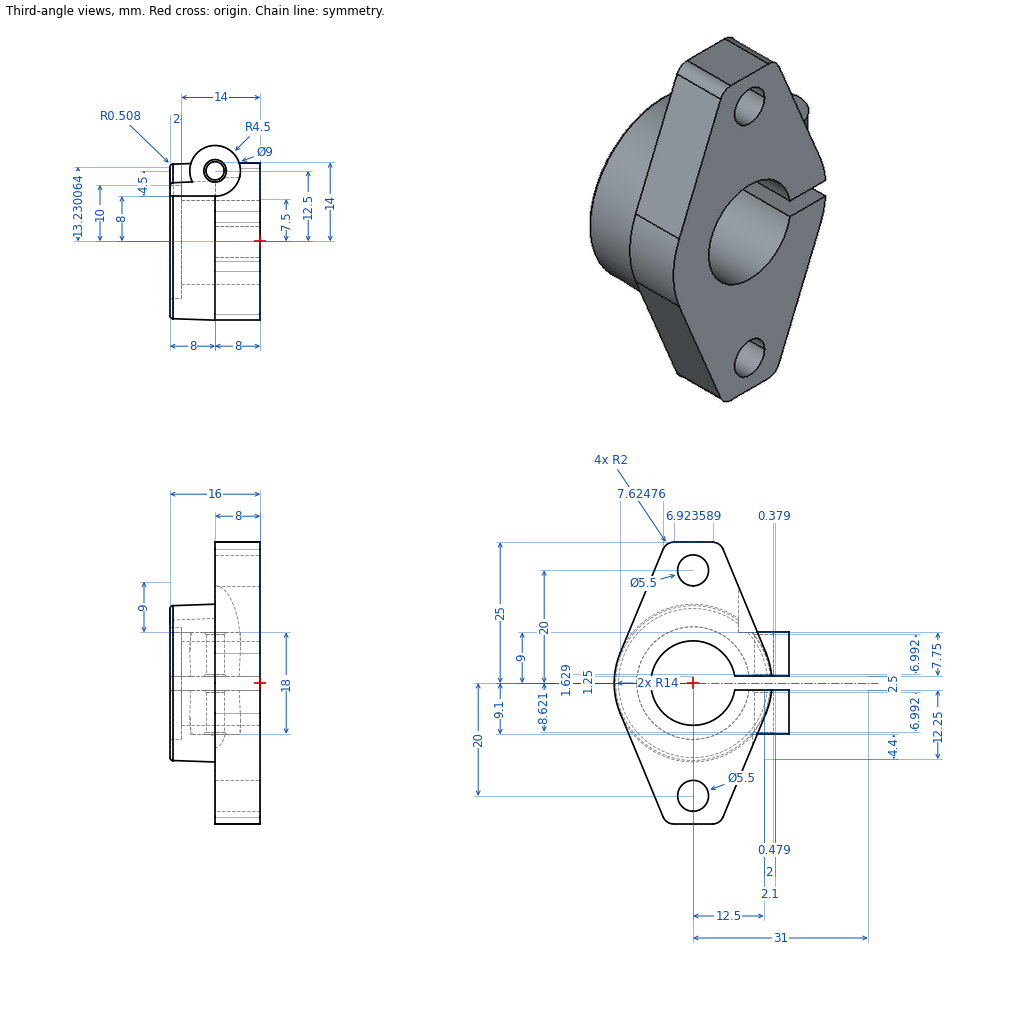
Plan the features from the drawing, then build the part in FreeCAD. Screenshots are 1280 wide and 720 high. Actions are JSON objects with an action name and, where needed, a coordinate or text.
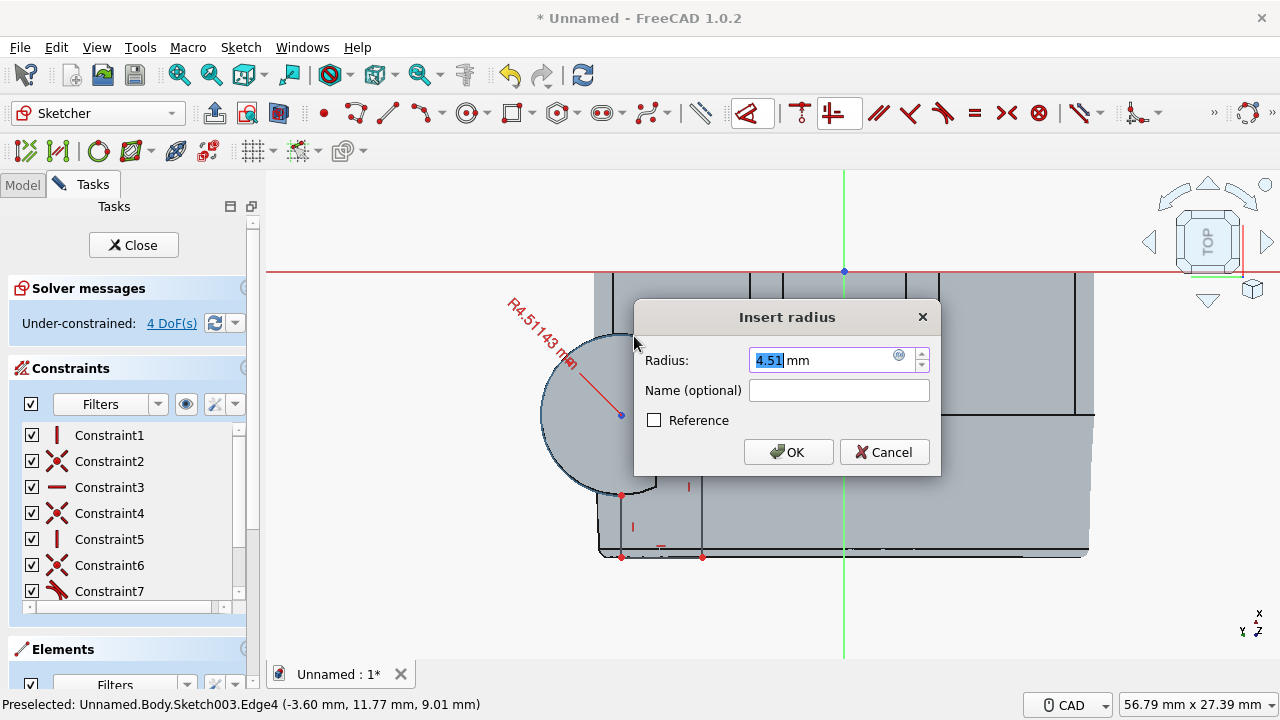
{"action": "type", "text": "4.5"}
{"action": "key", "text": "Return"}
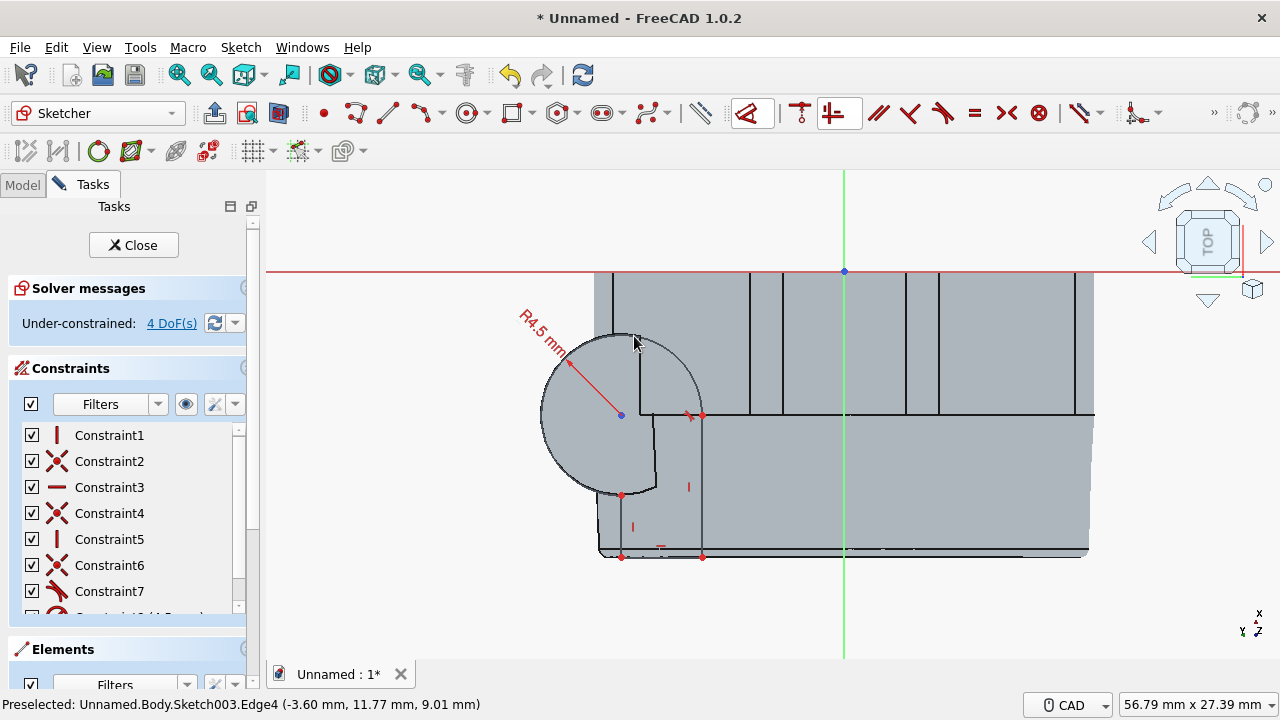
{"action": "left_click", "coordinate": [702, 515]}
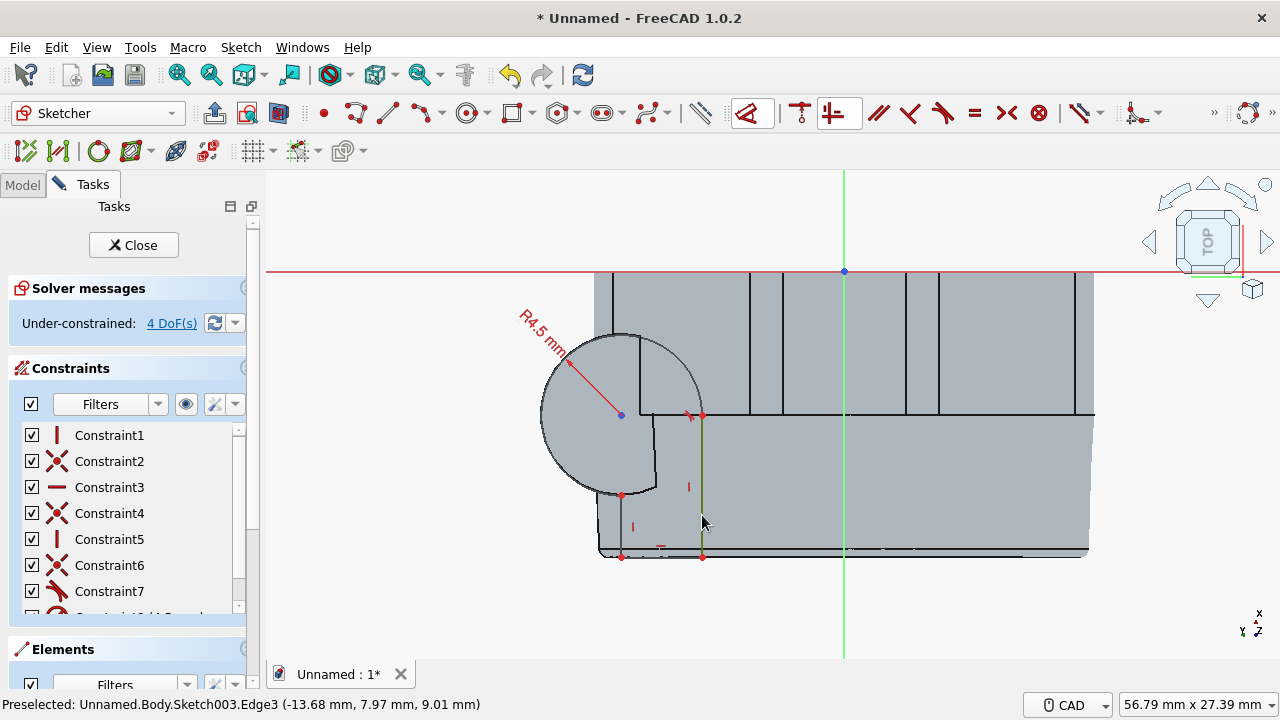
{"action": "left_click", "coordinate": [768, 114]}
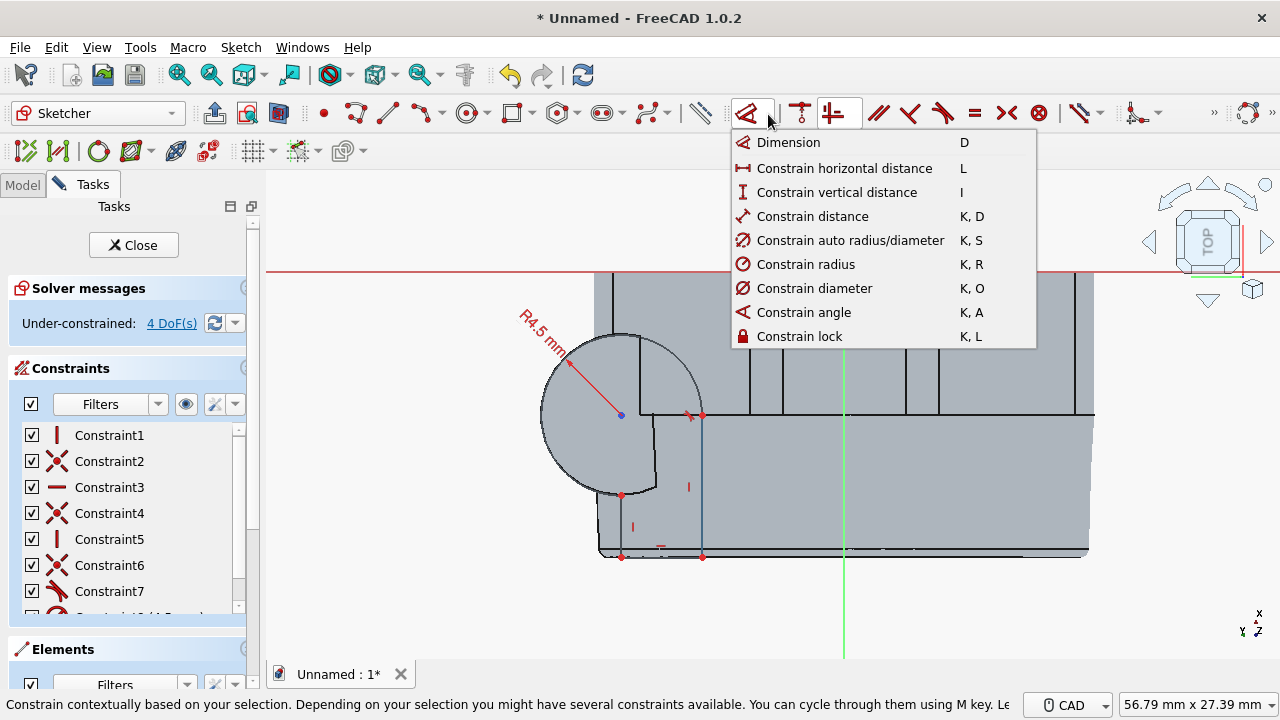
{"action": "left_click", "coordinate": [884, 192]}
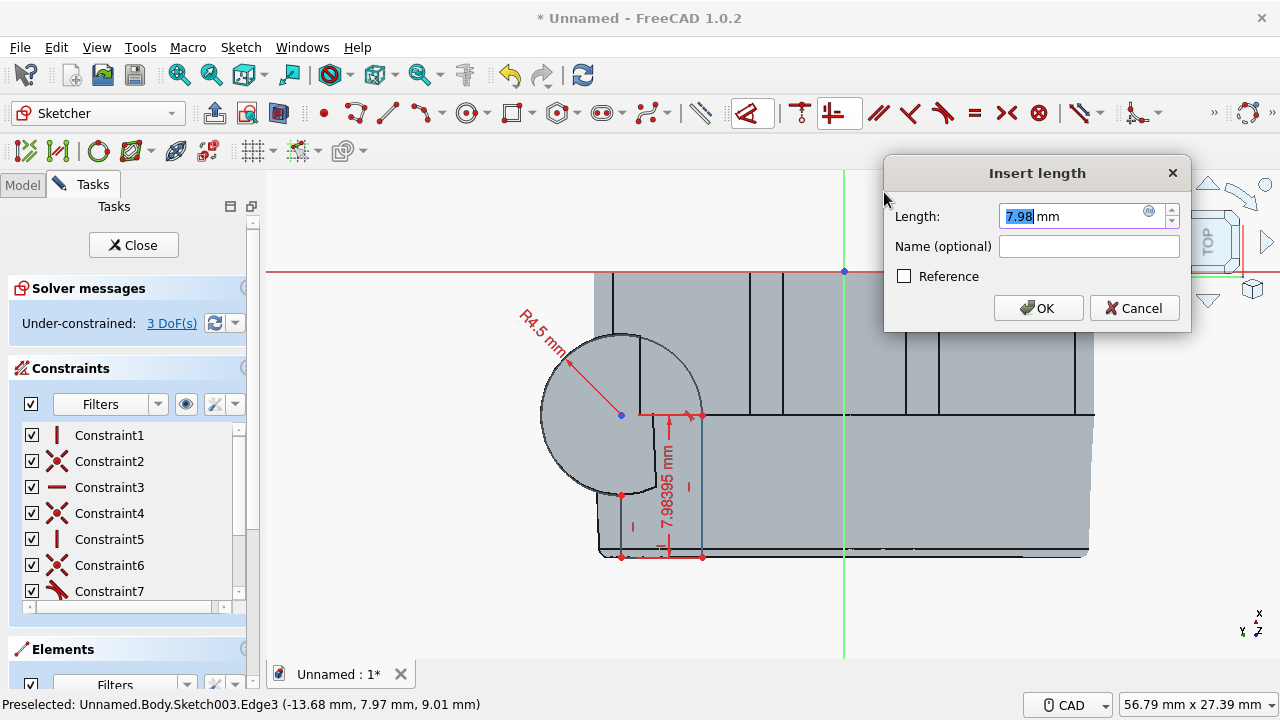
{"action": "type", "text": "8"}
{"action": "key", "text": "Return"}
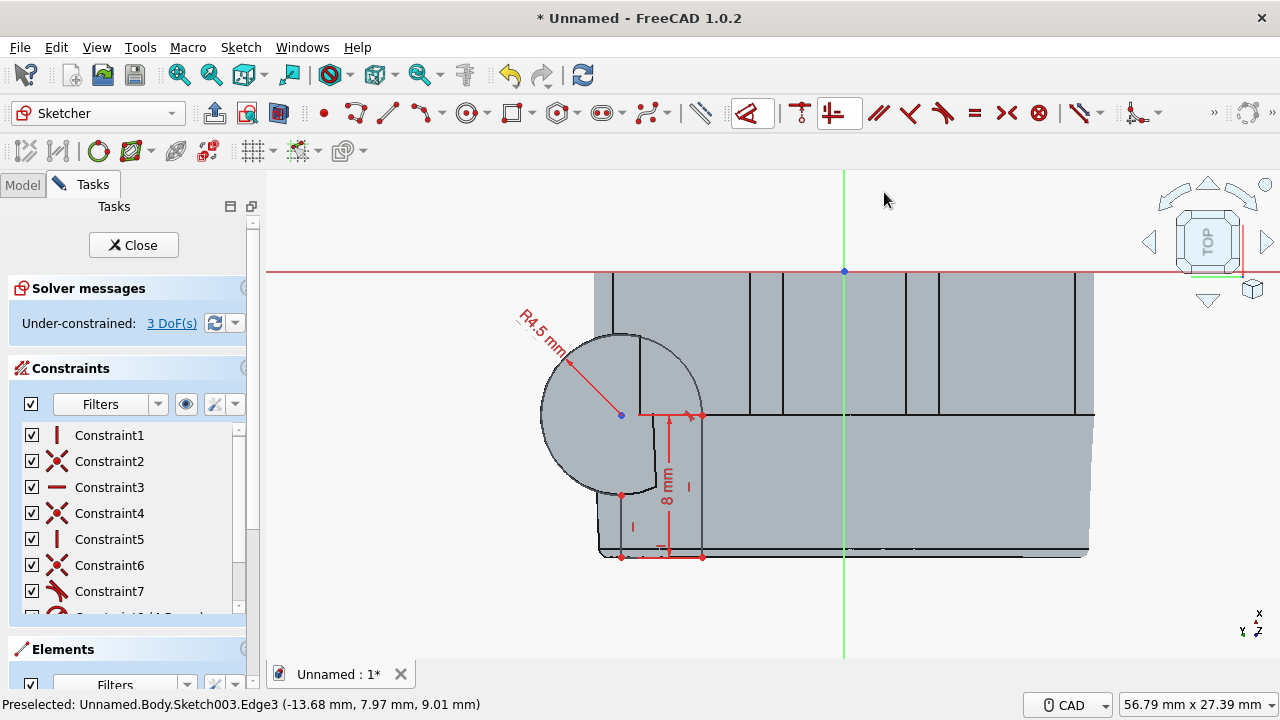
{"action": "left_click", "coordinate": [702, 558]}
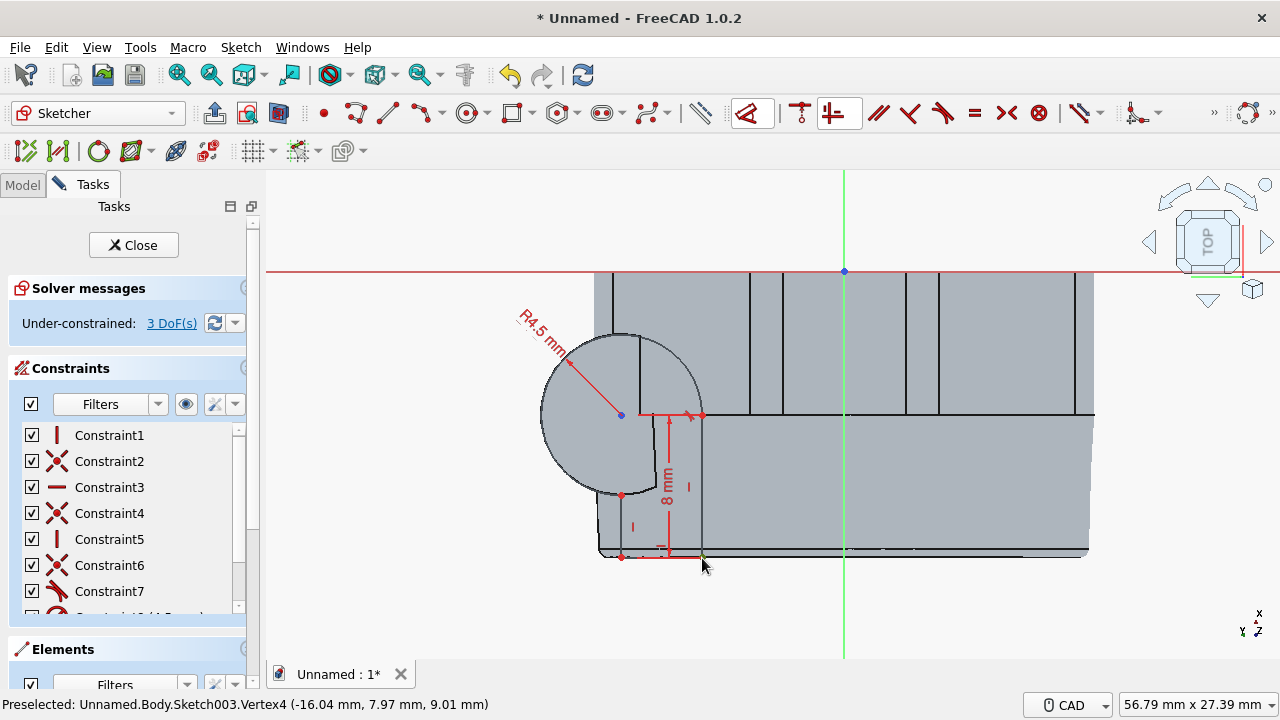
{"action": "left_click", "coordinate": [768, 114]}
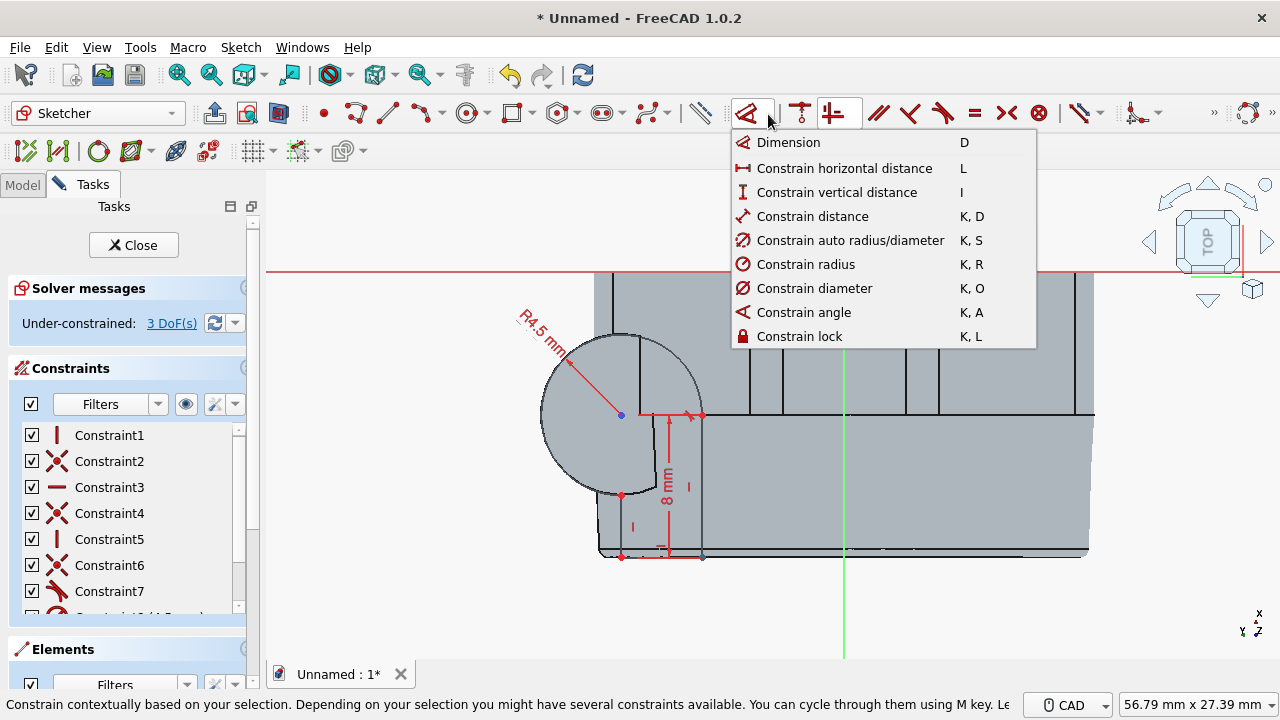
{"action": "left_click", "coordinate": [884, 168]}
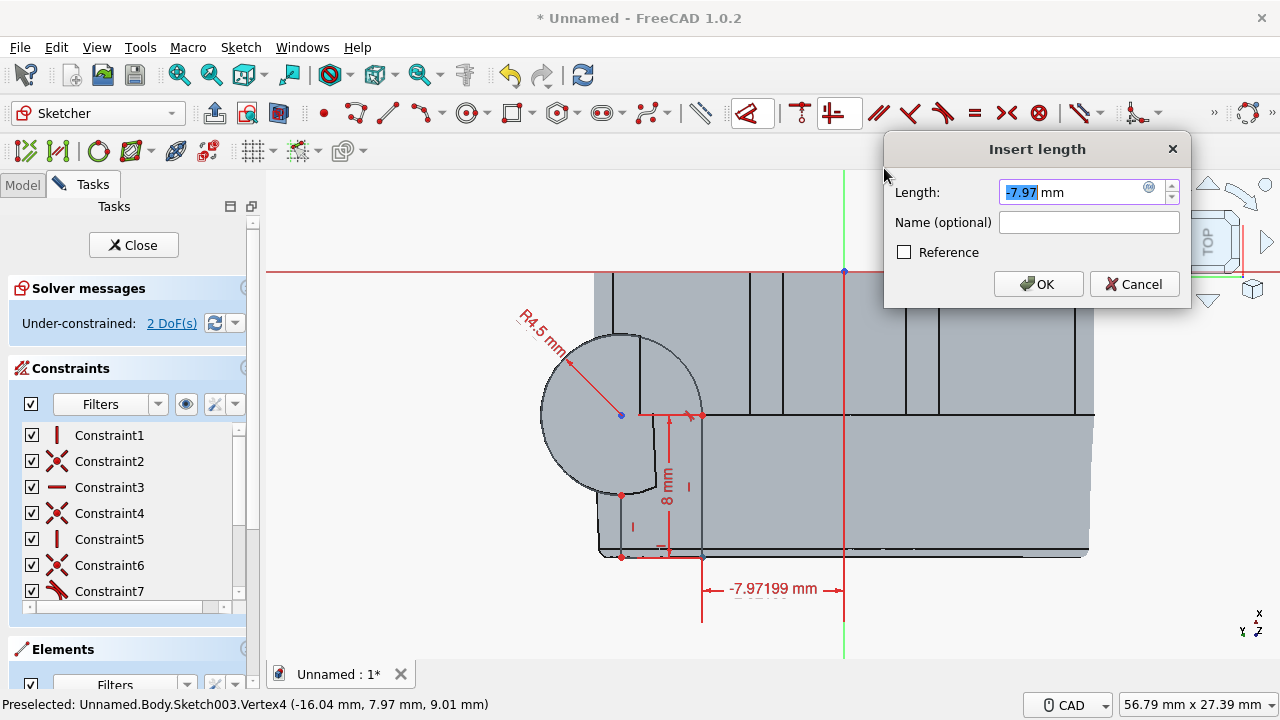
{"action": "type", "text": "-8"}
{"action": "key", "text": "Return"}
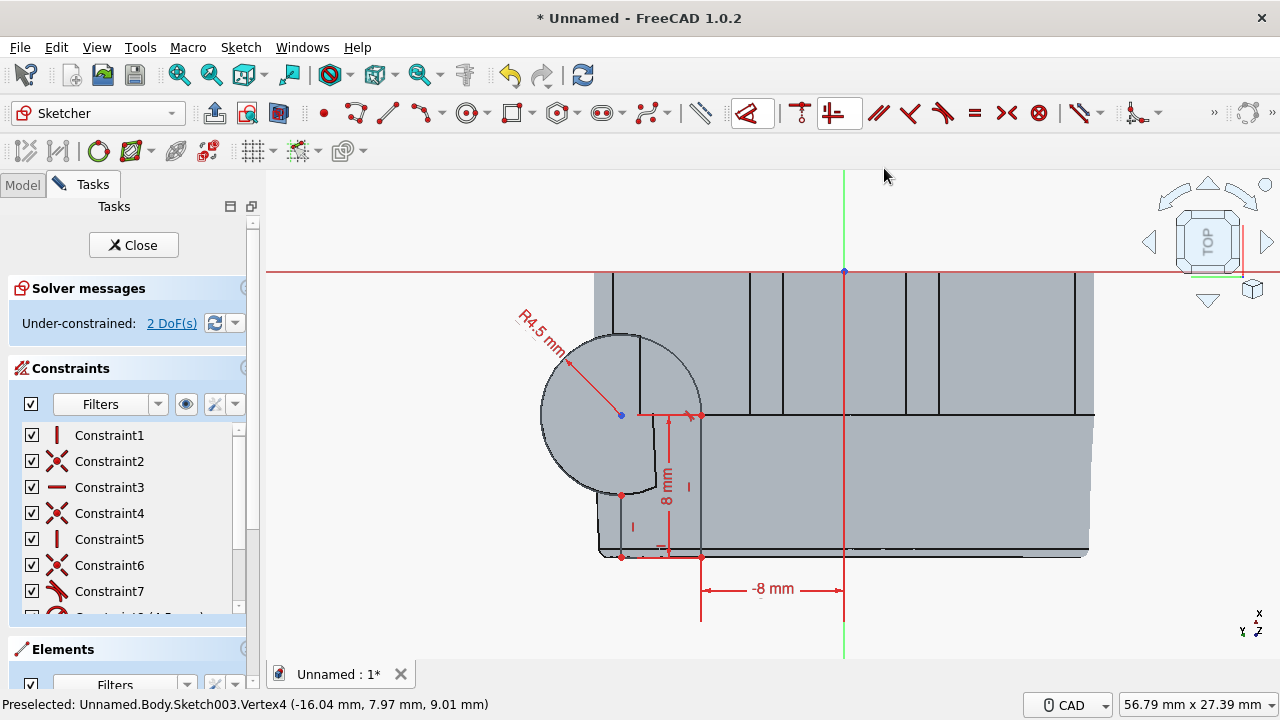
{"action": "left_click", "coordinate": [702, 415]}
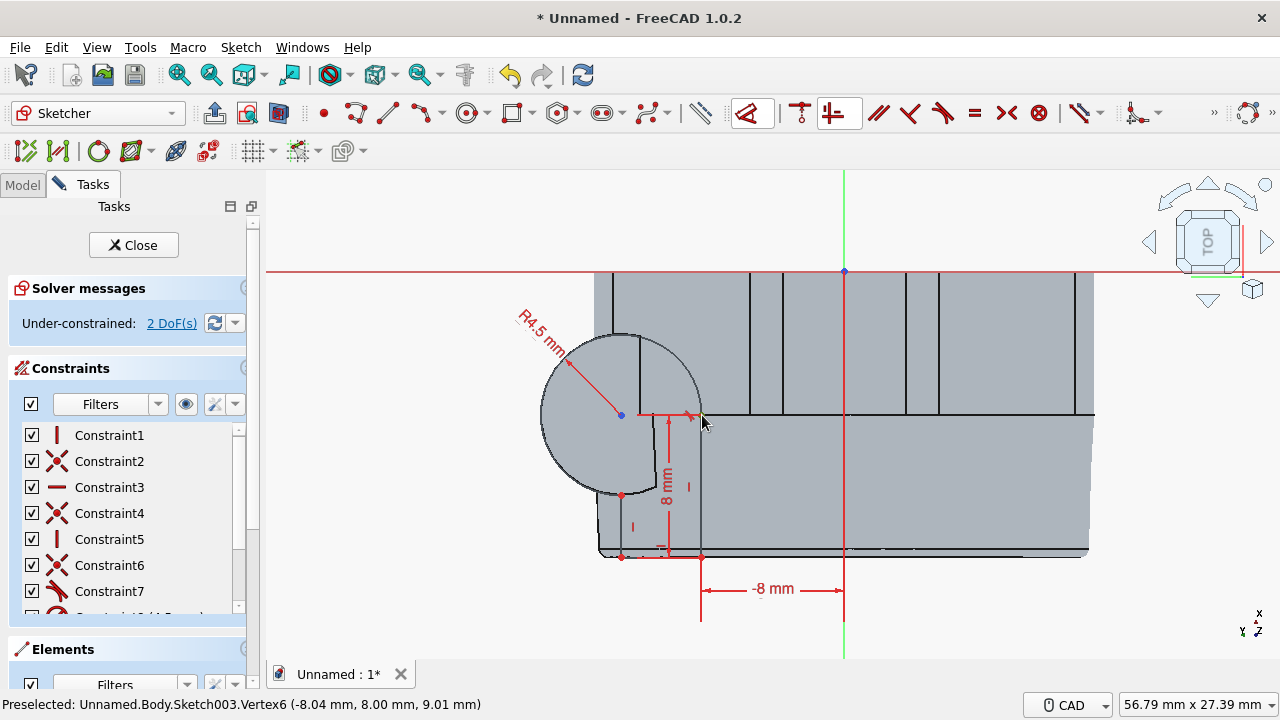
{"action": "key", "text": "i"}